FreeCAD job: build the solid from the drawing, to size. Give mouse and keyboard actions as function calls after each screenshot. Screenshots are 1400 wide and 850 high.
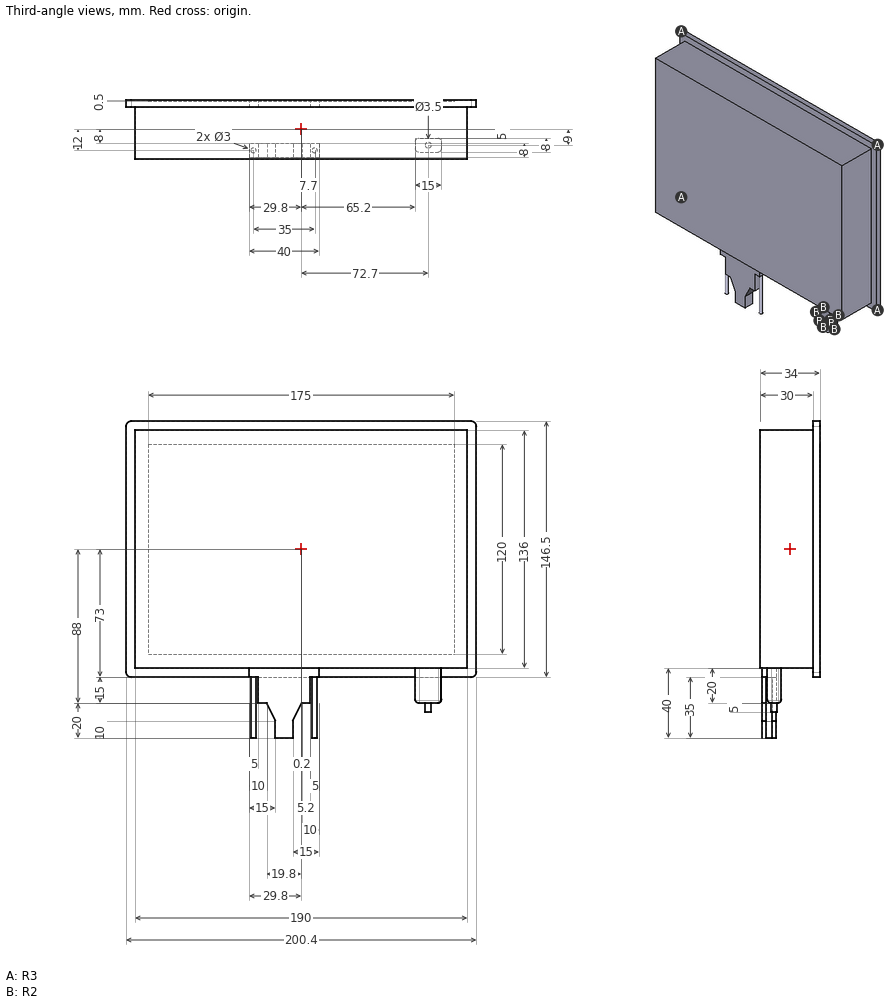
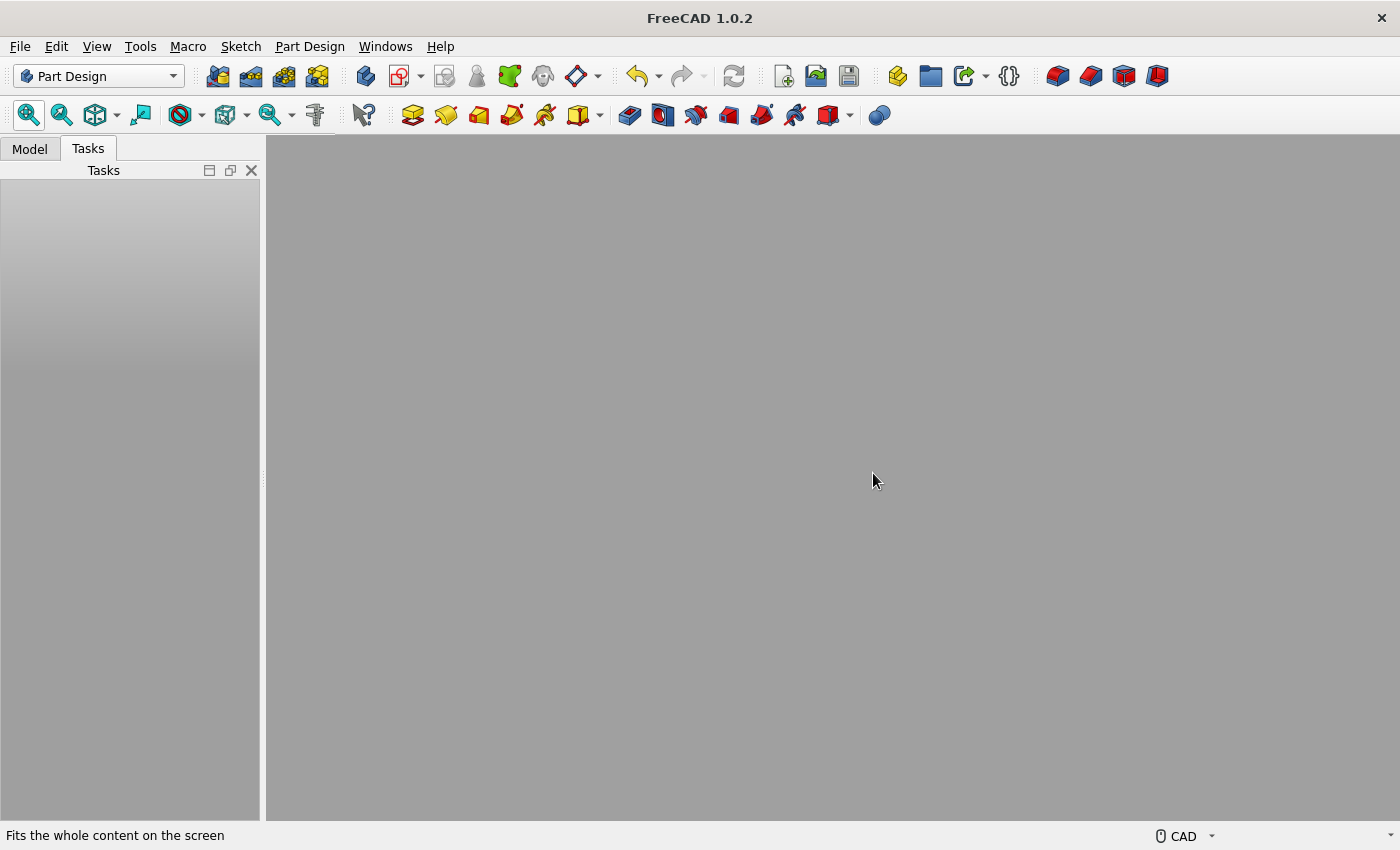
click(783, 76)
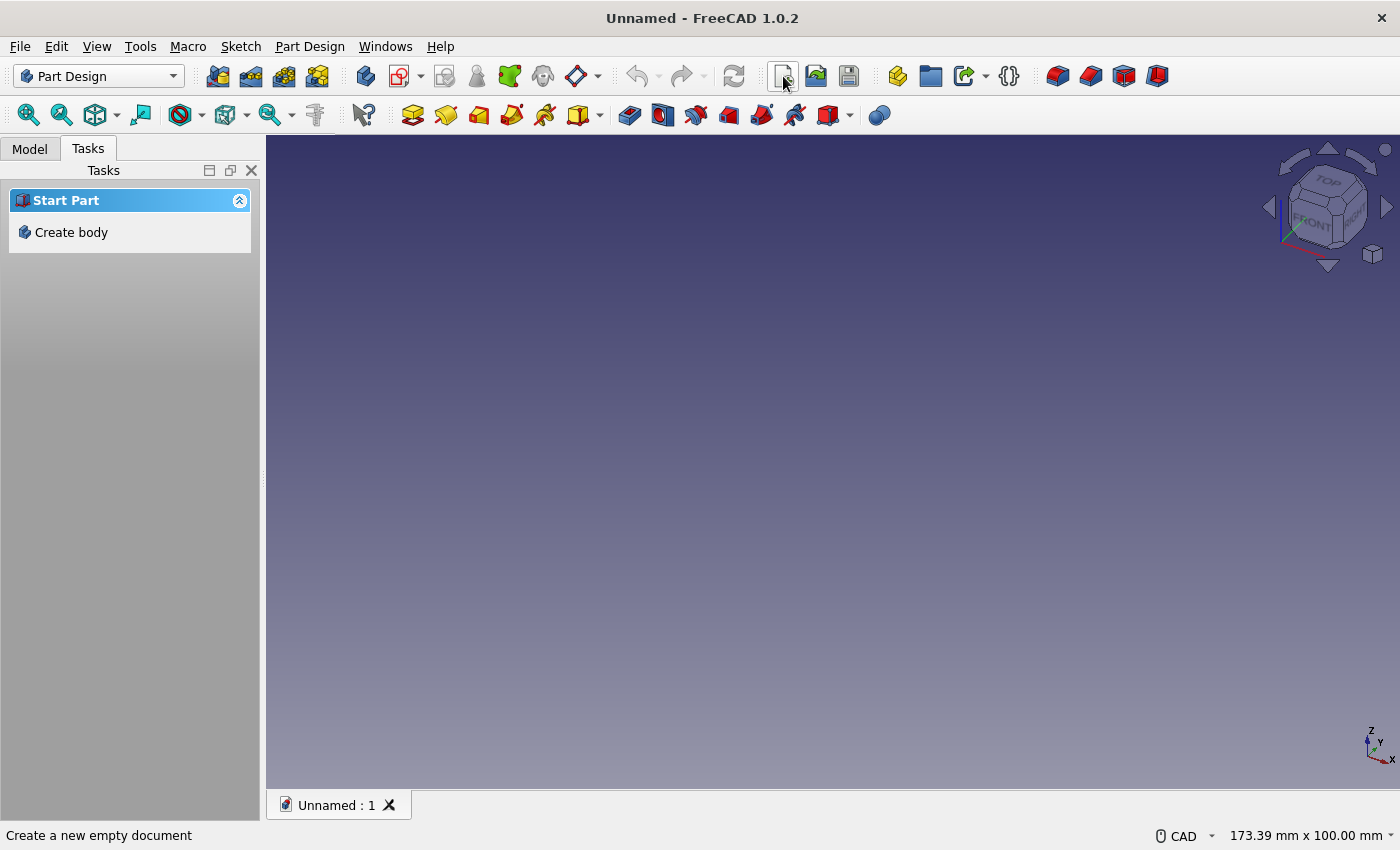
click(398, 76)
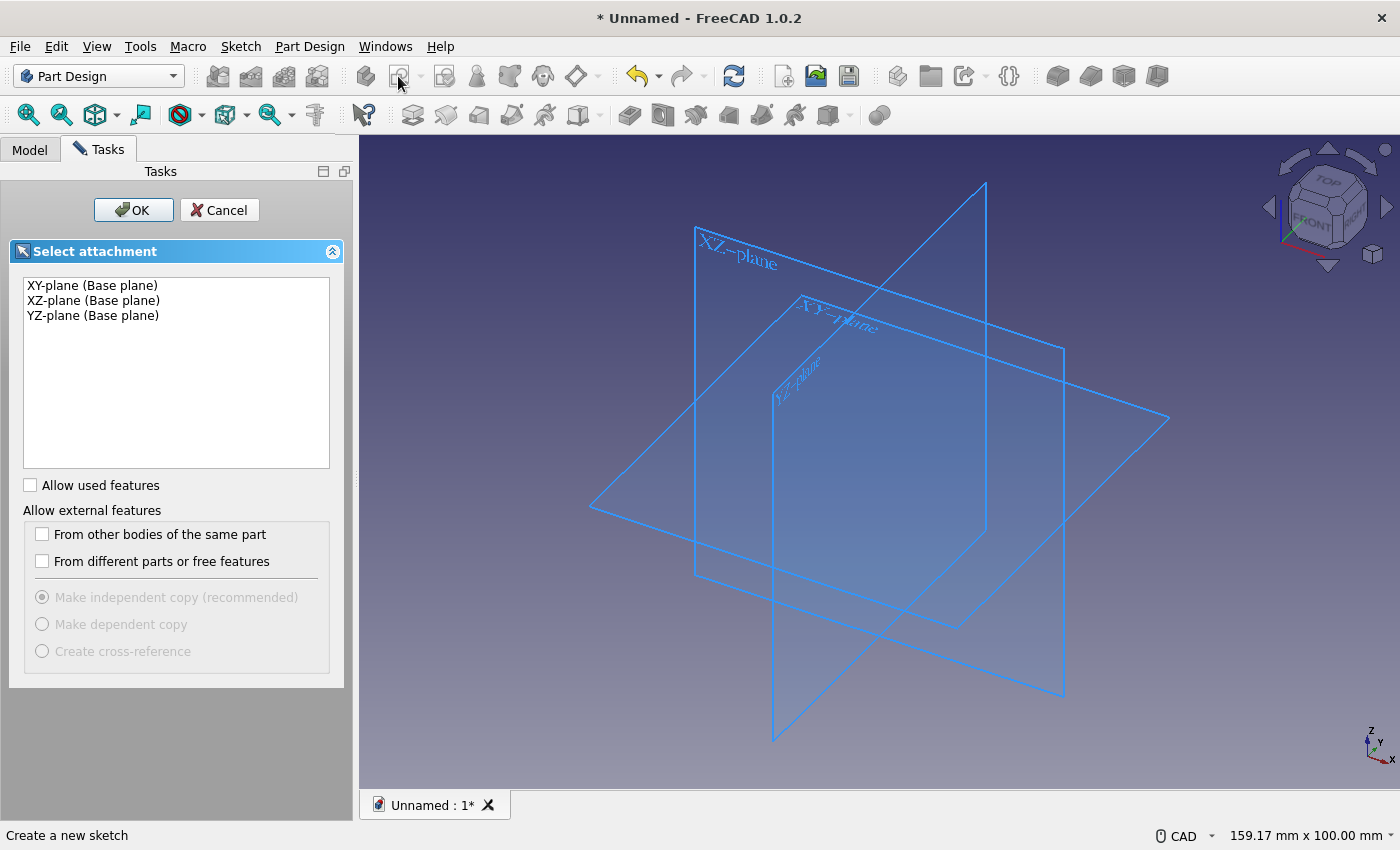
click(84, 300)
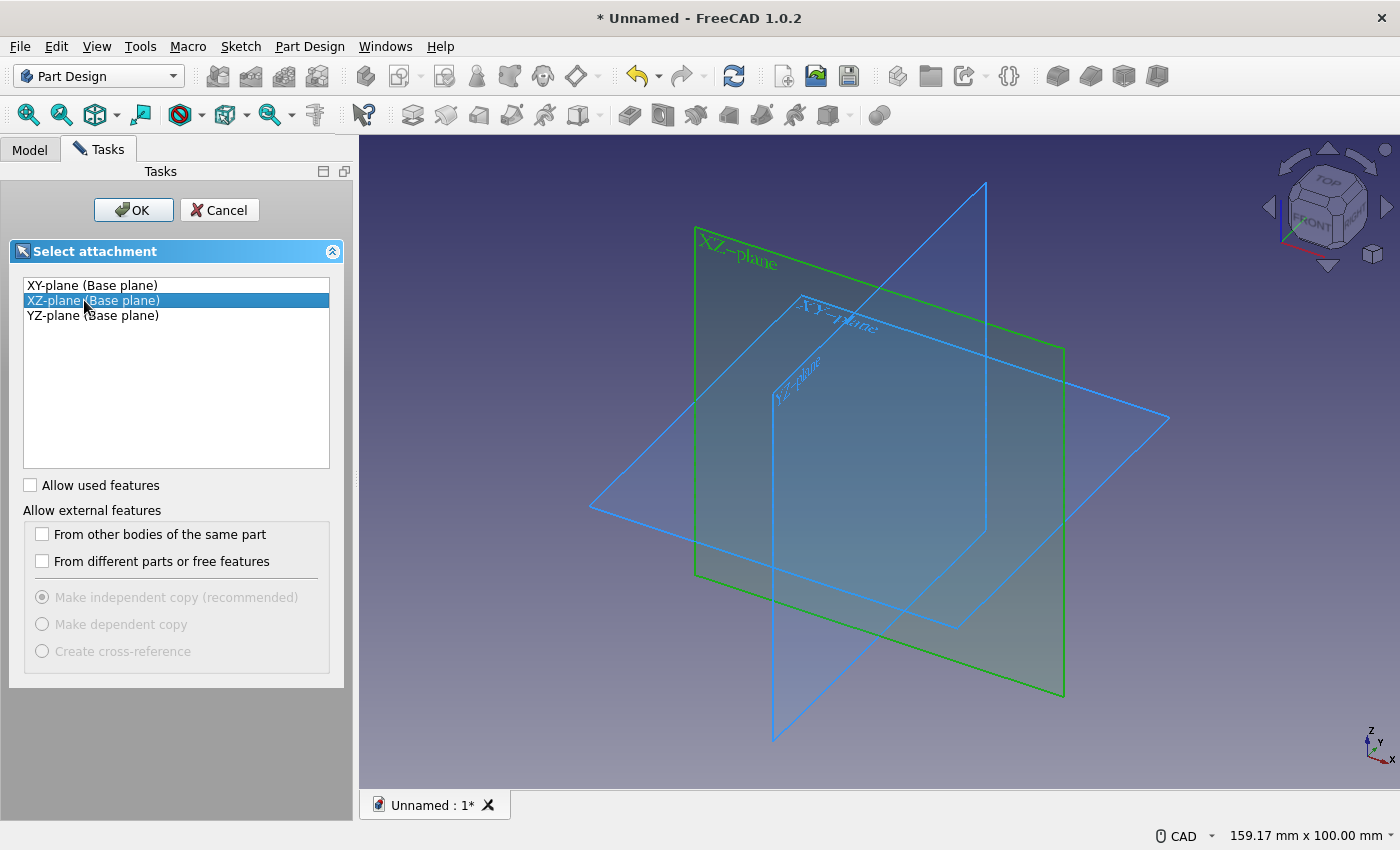
click(134, 210)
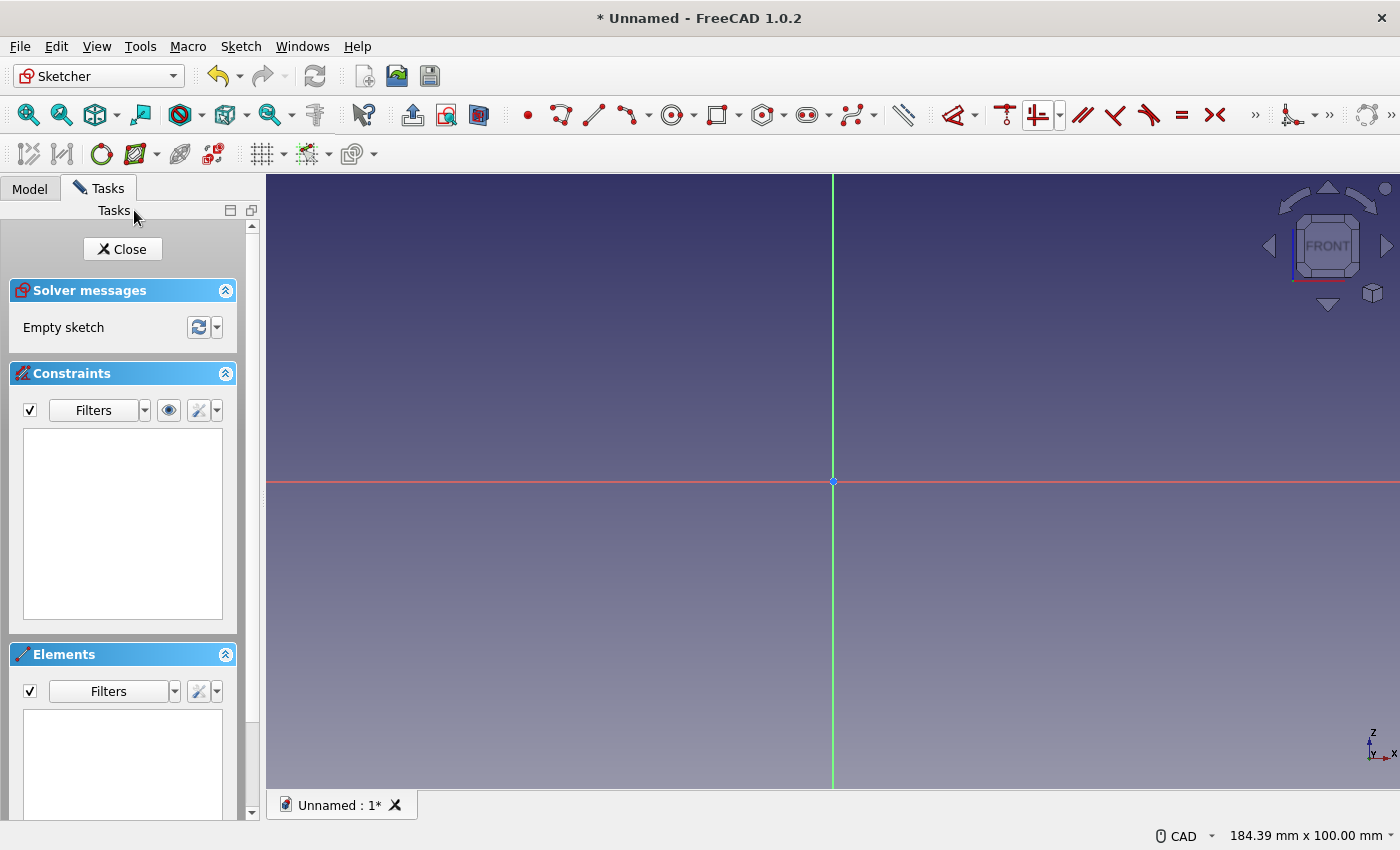
scroll(709, 482, down, 4)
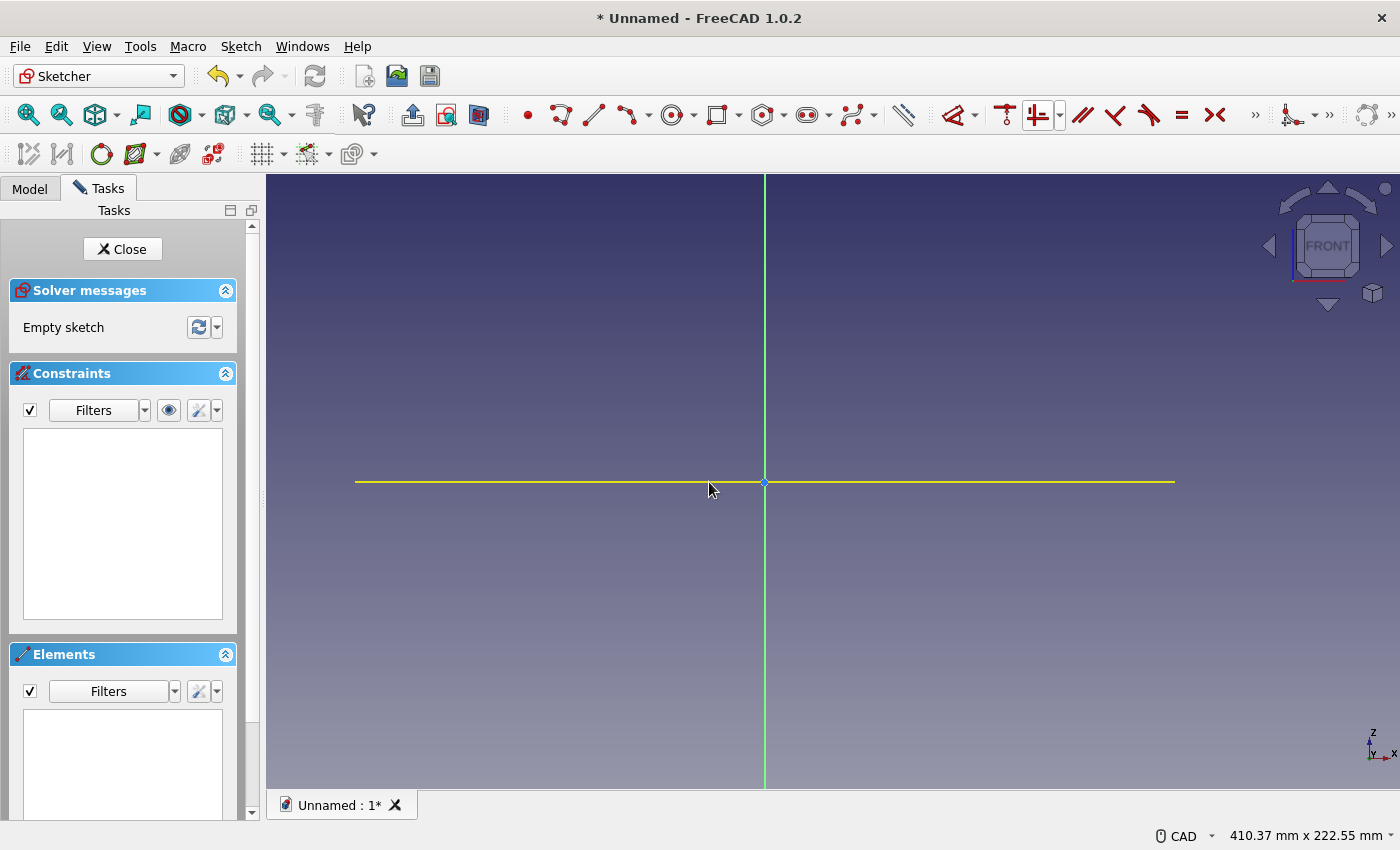
key(g)
key(v)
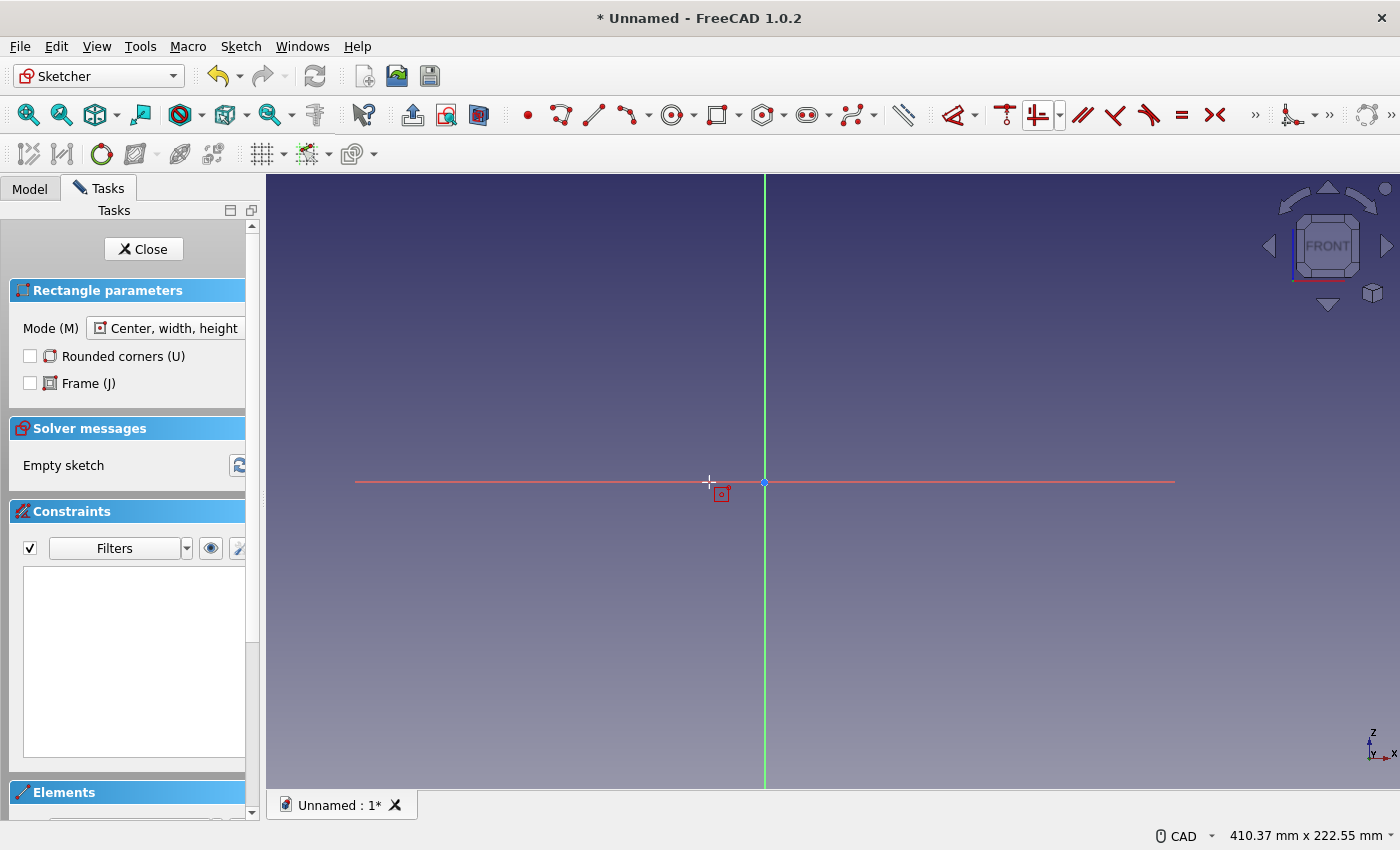
click(765, 482)
move(1042, 280)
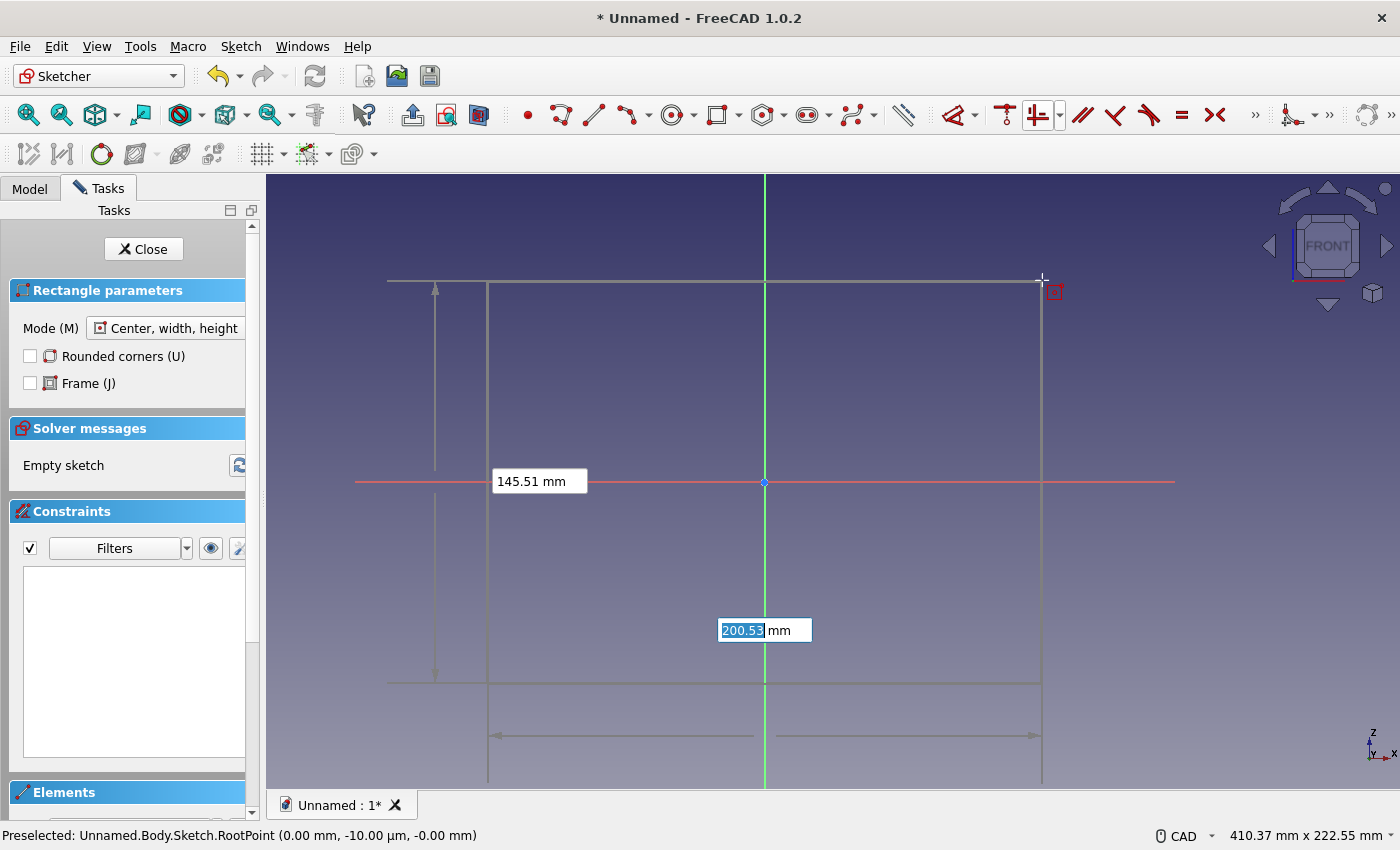
text(200.4)
key(Tab)
text(146.5)
key(Return)
key(Escape)